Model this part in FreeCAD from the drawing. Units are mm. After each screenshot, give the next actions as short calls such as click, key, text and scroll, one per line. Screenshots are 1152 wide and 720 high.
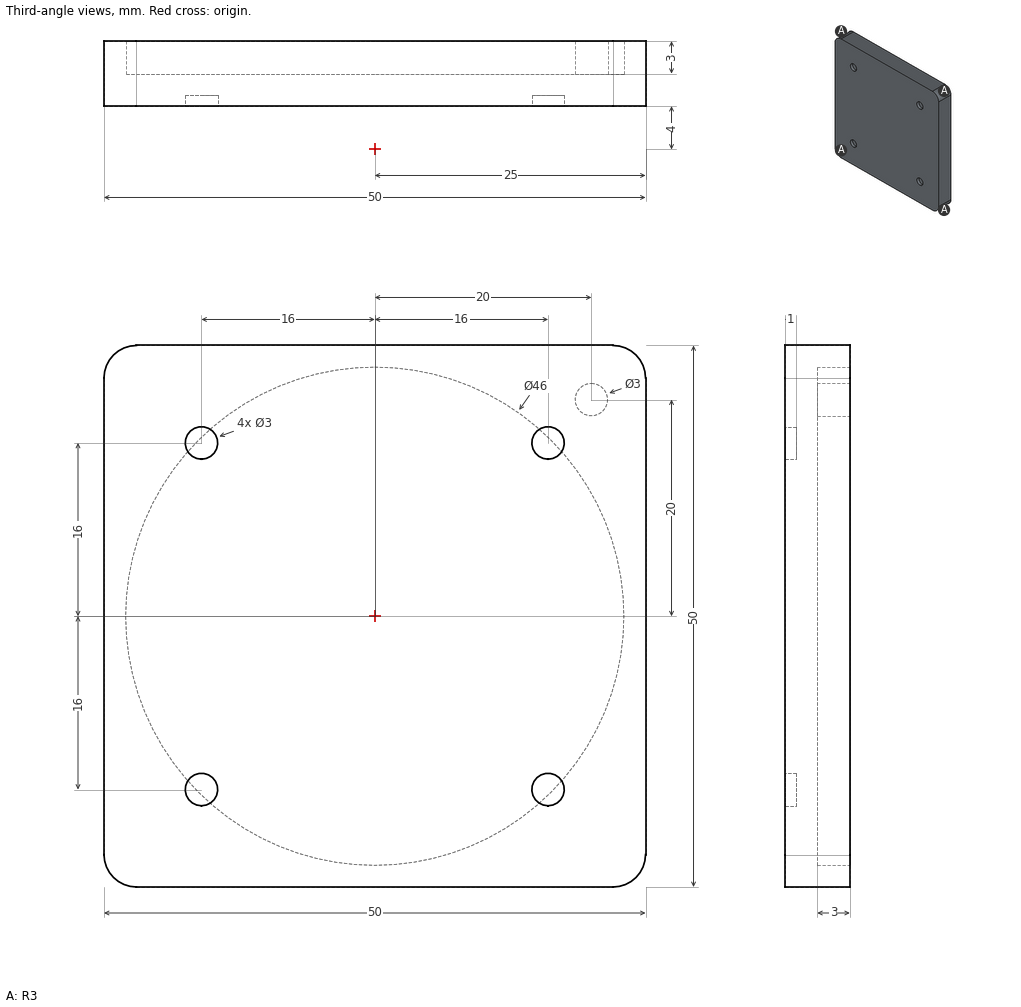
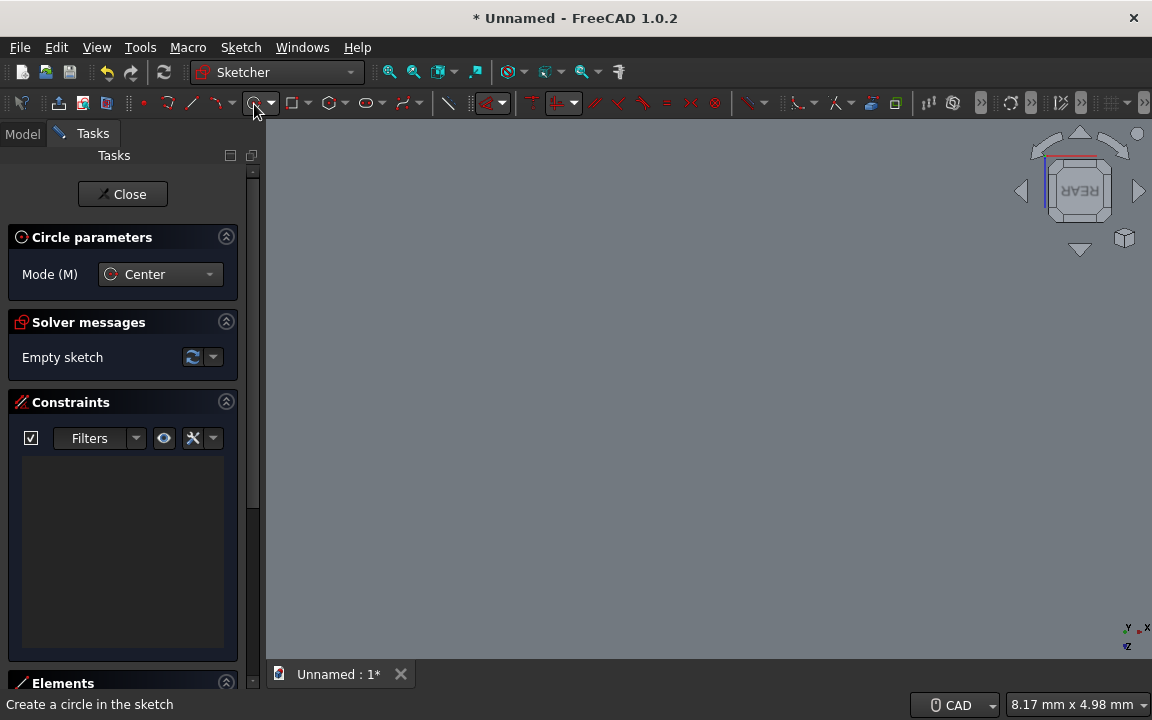
click(633, 369)
click(748, 254)
key(Escape)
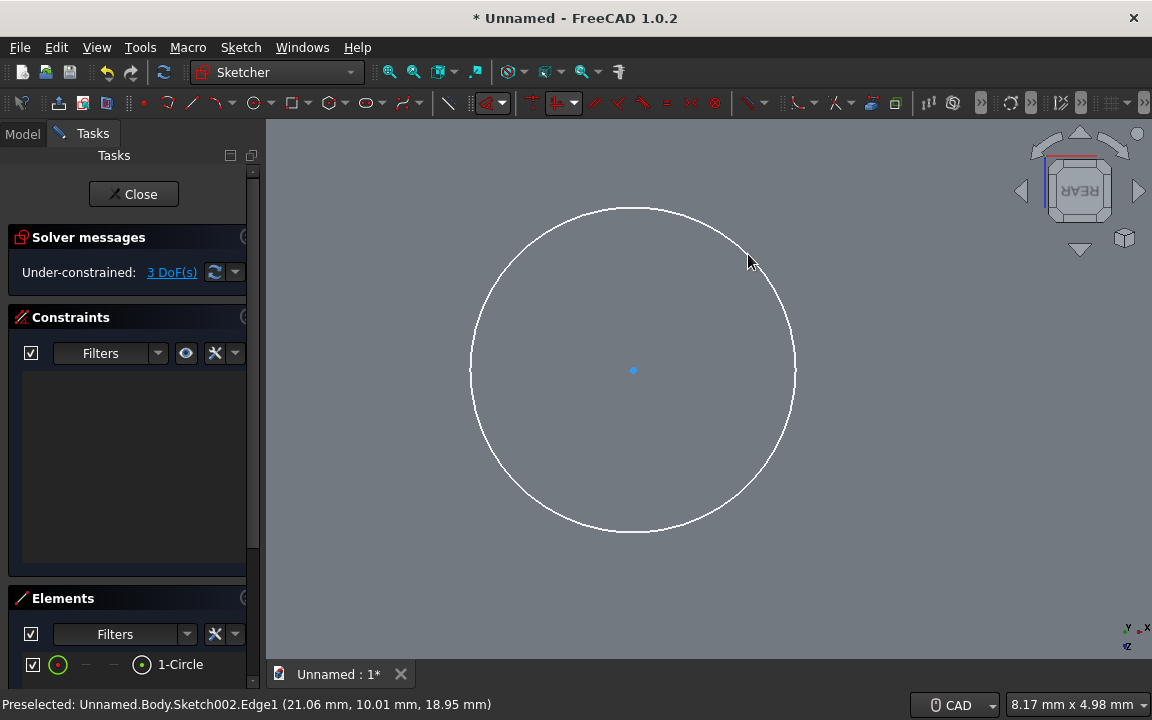
click(748, 255)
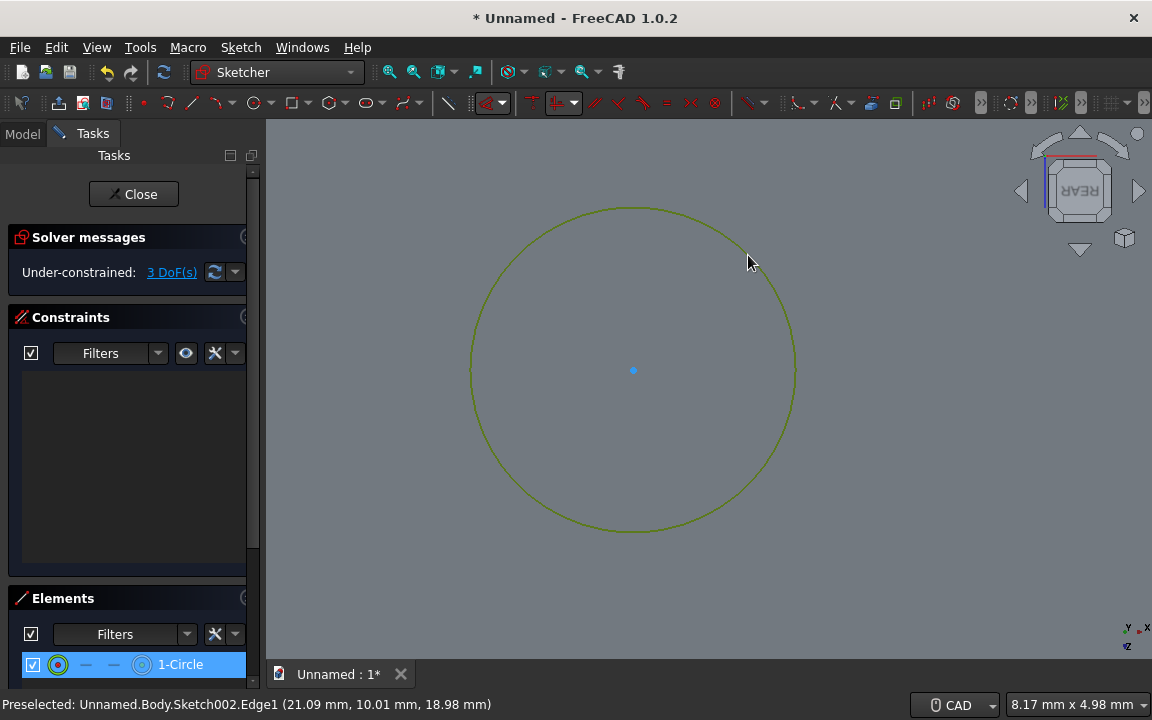
click(504, 104)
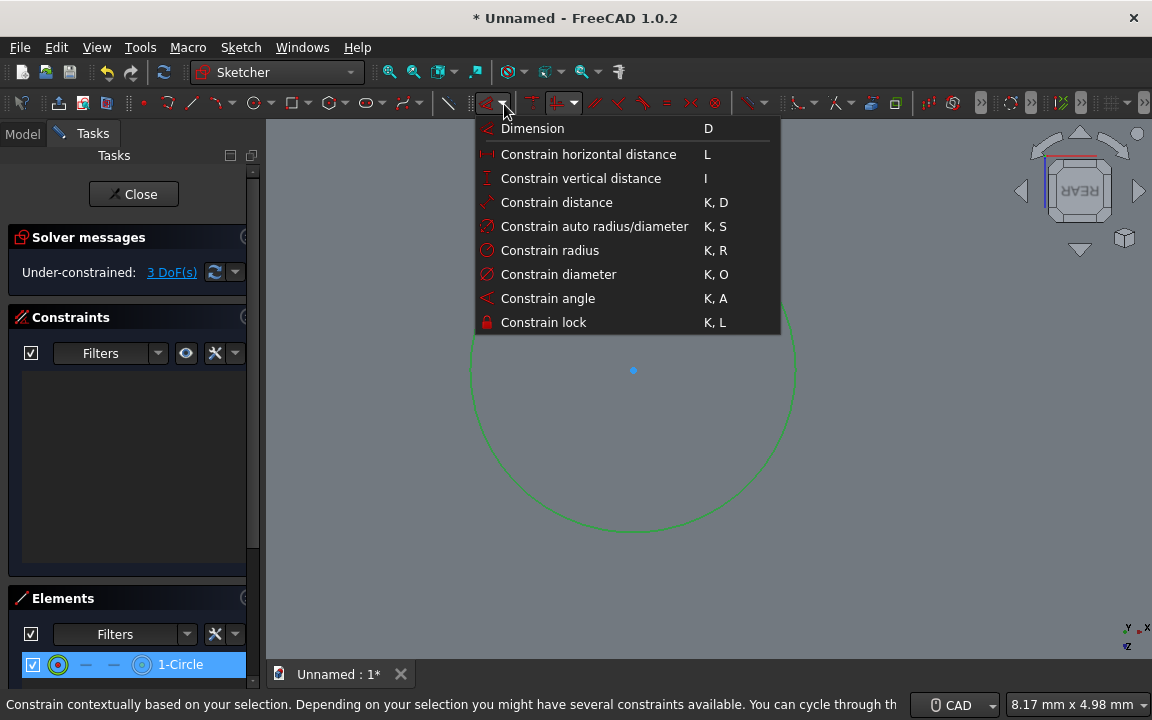
click(628, 274)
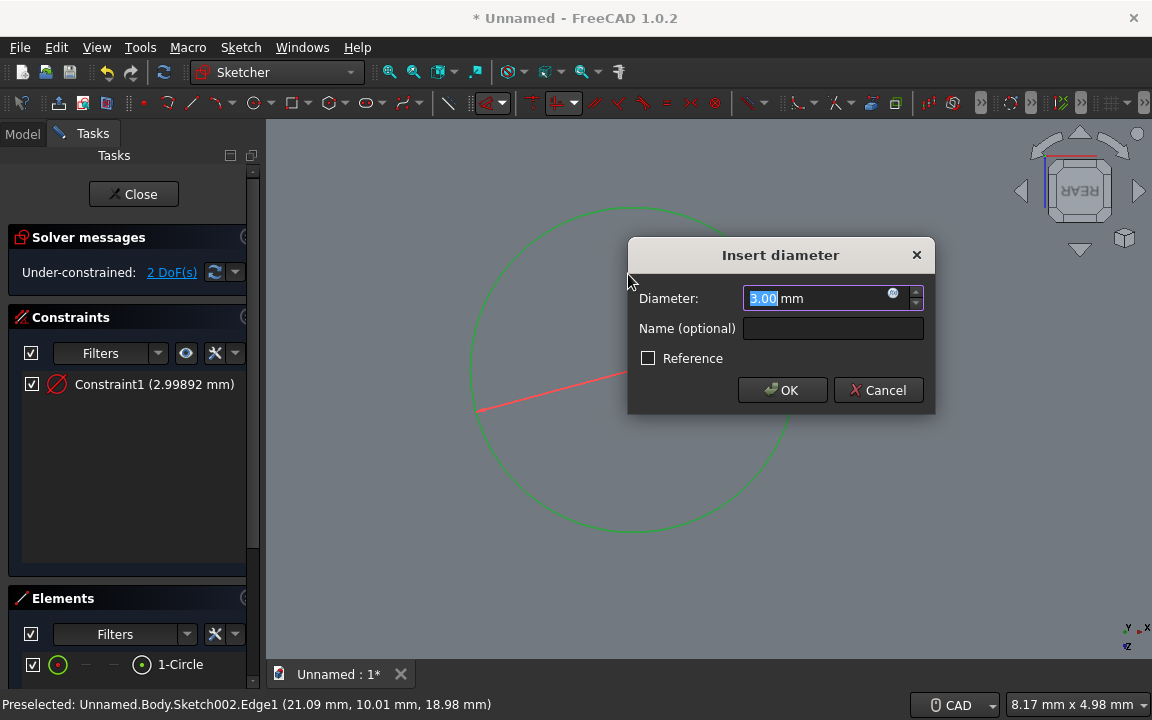
text(3)
key(Return)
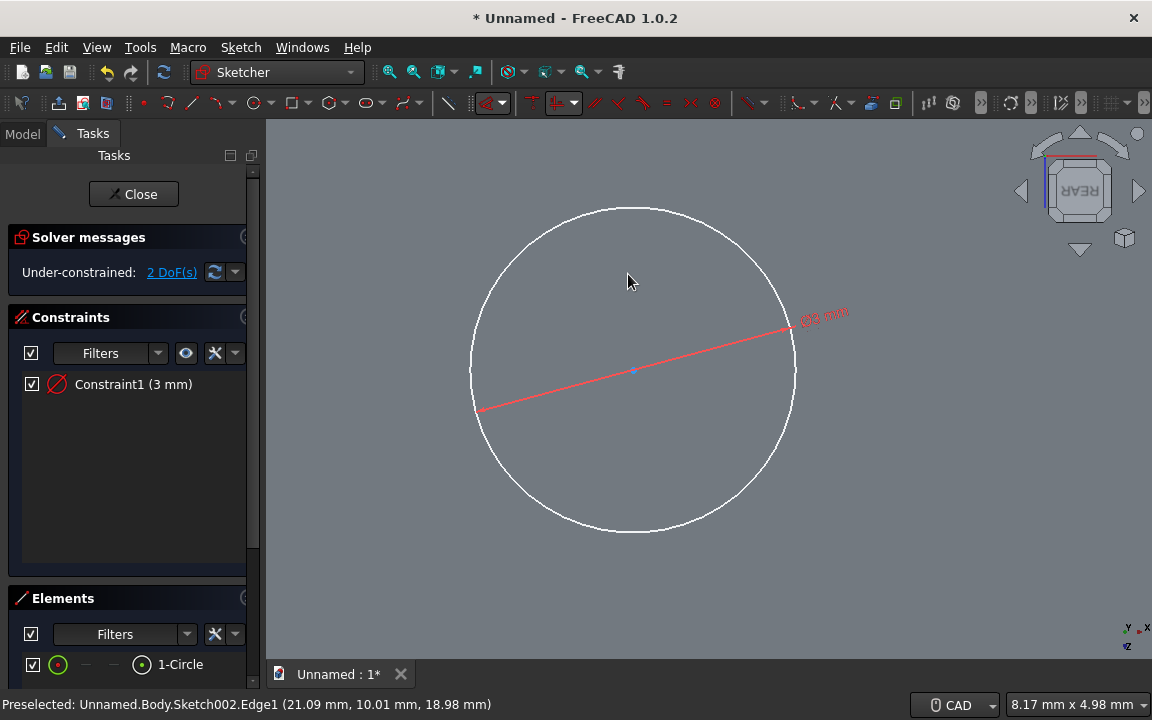
click(633, 370)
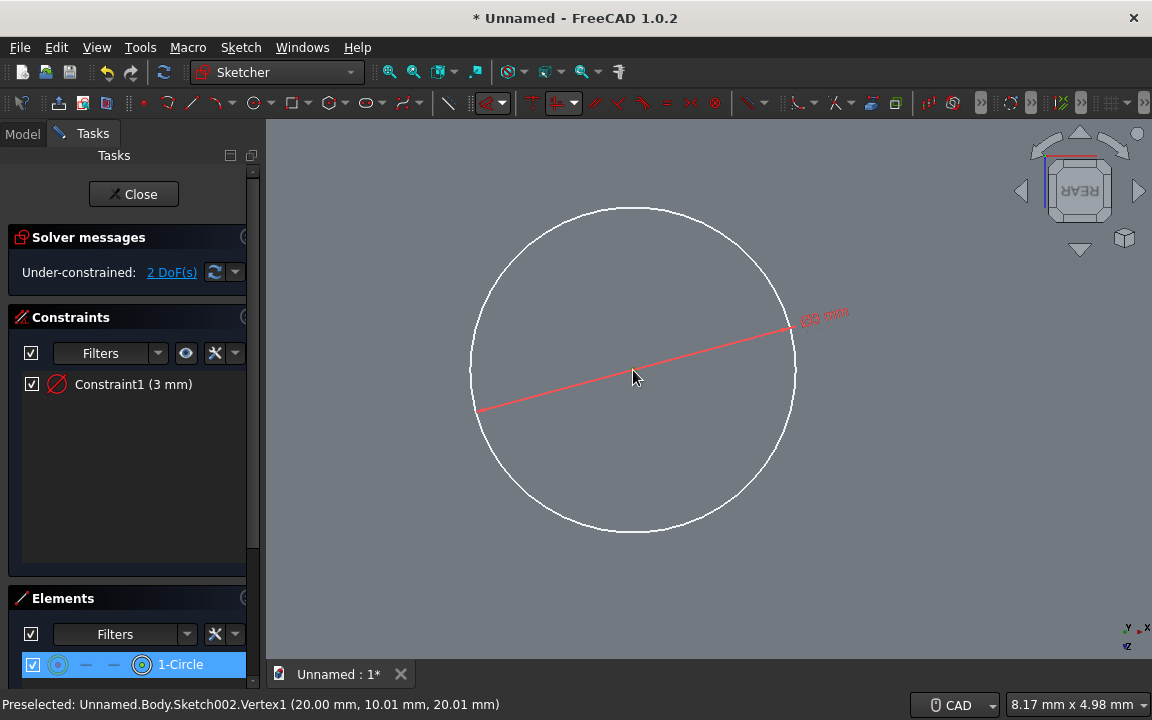
click(504, 104)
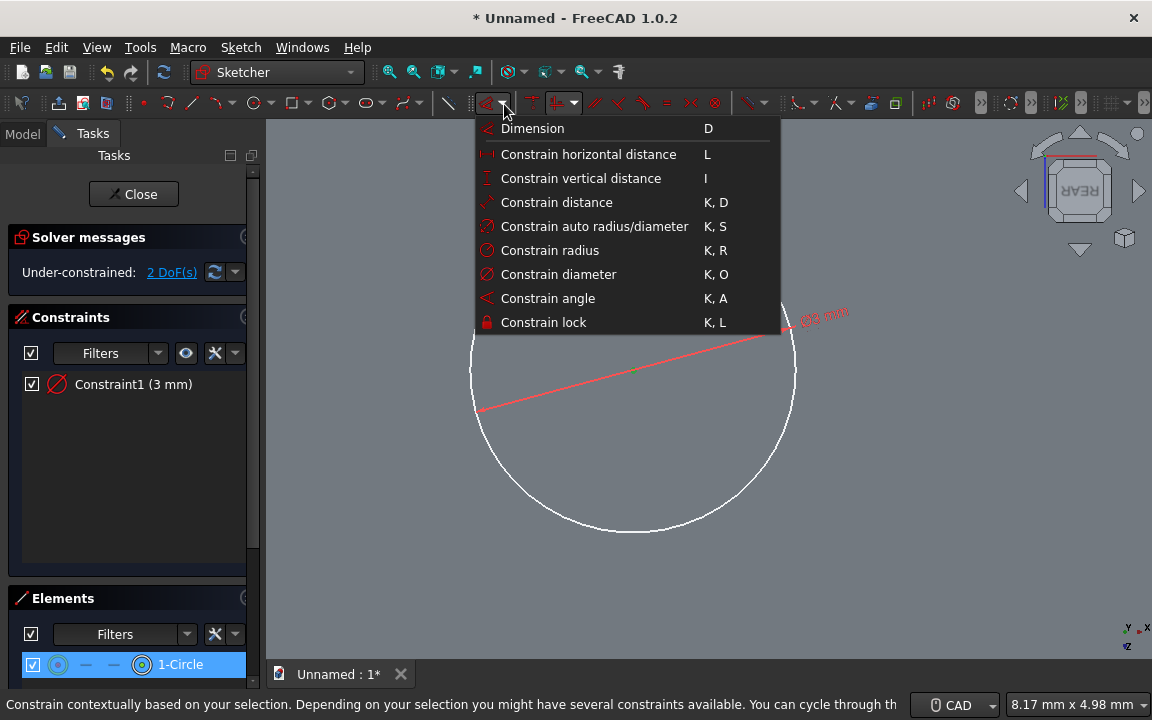
click(628, 154)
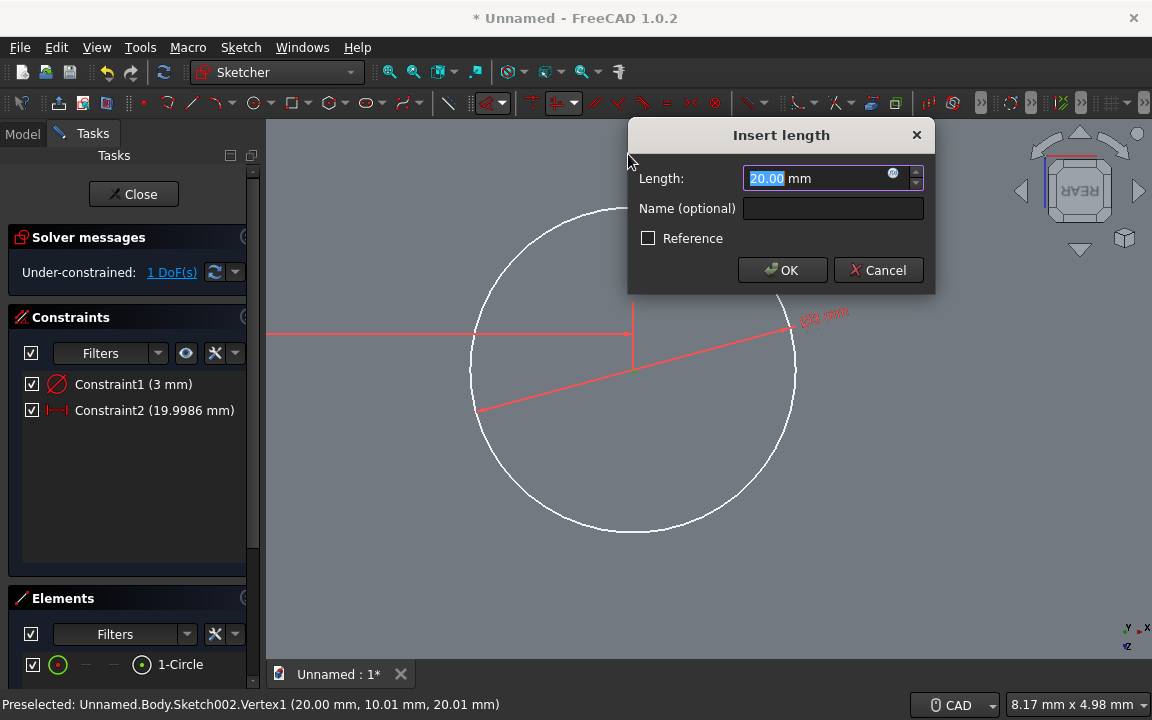
text(20)
key(Return)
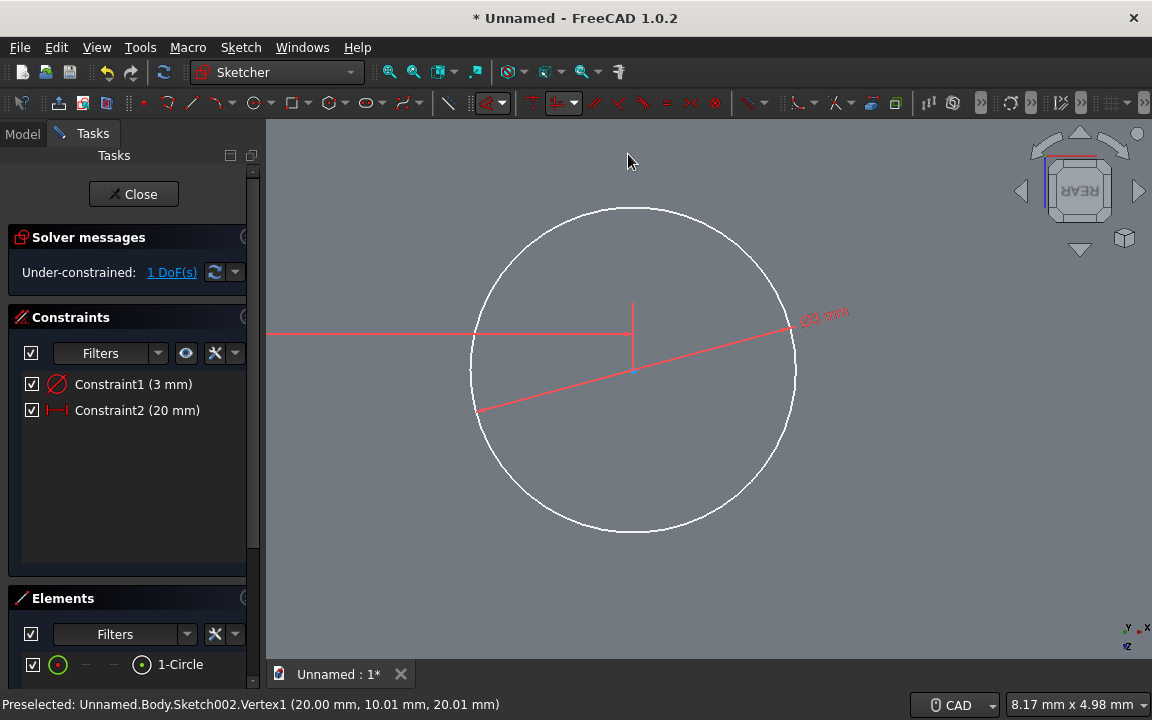
click(633, 370)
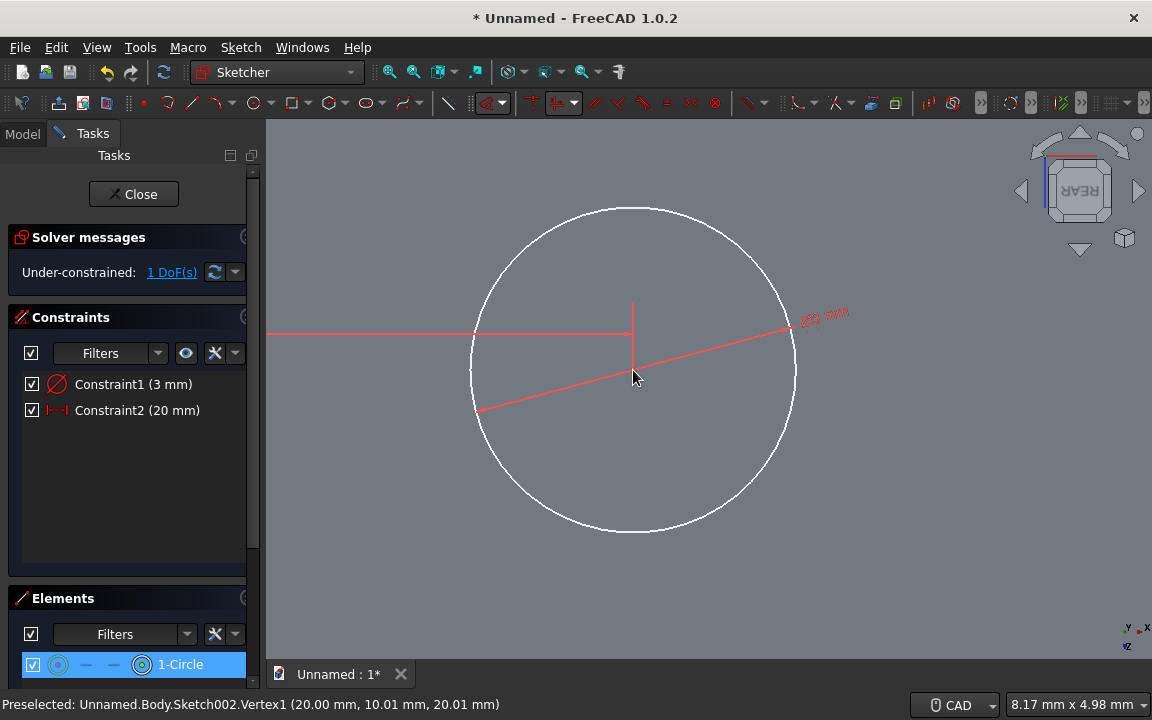
key(i)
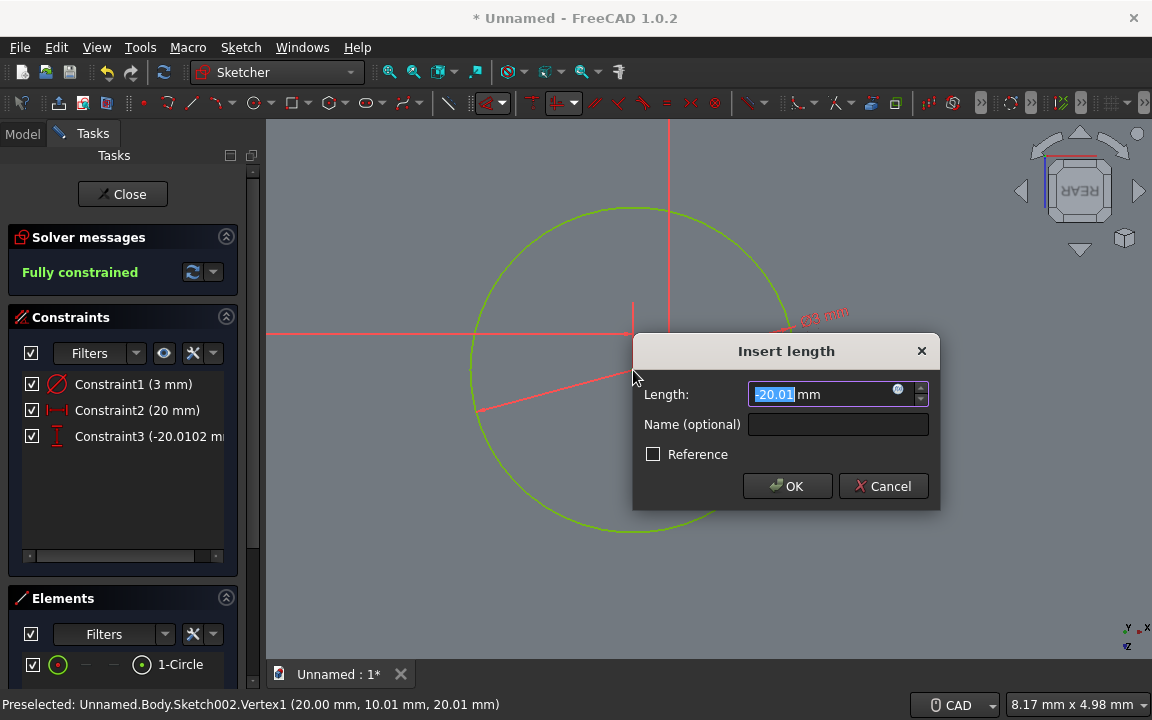
text(-20)
key(Return)